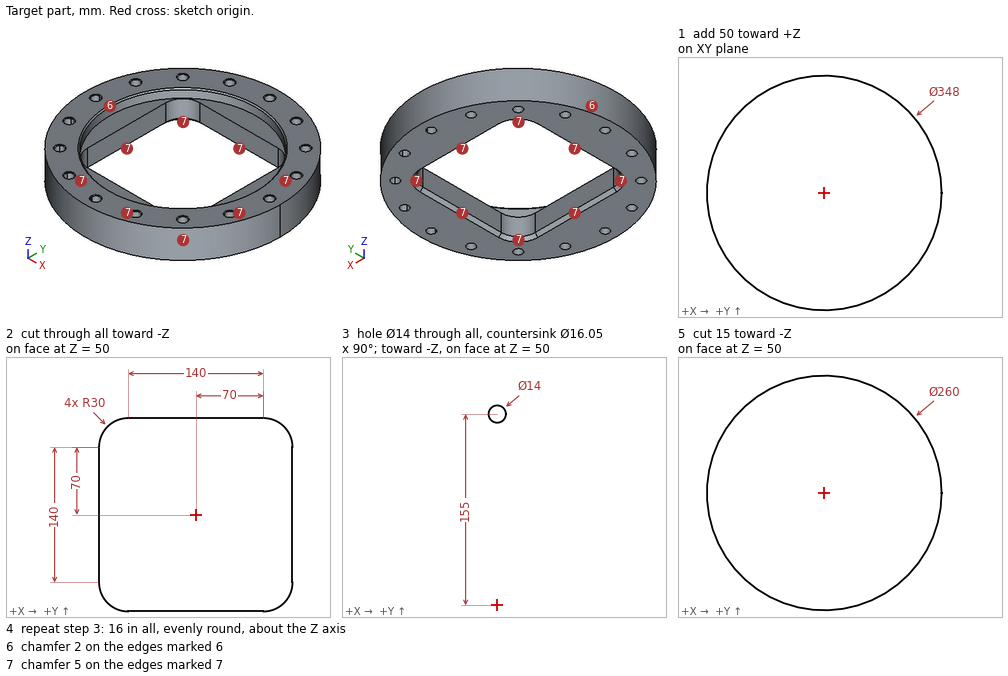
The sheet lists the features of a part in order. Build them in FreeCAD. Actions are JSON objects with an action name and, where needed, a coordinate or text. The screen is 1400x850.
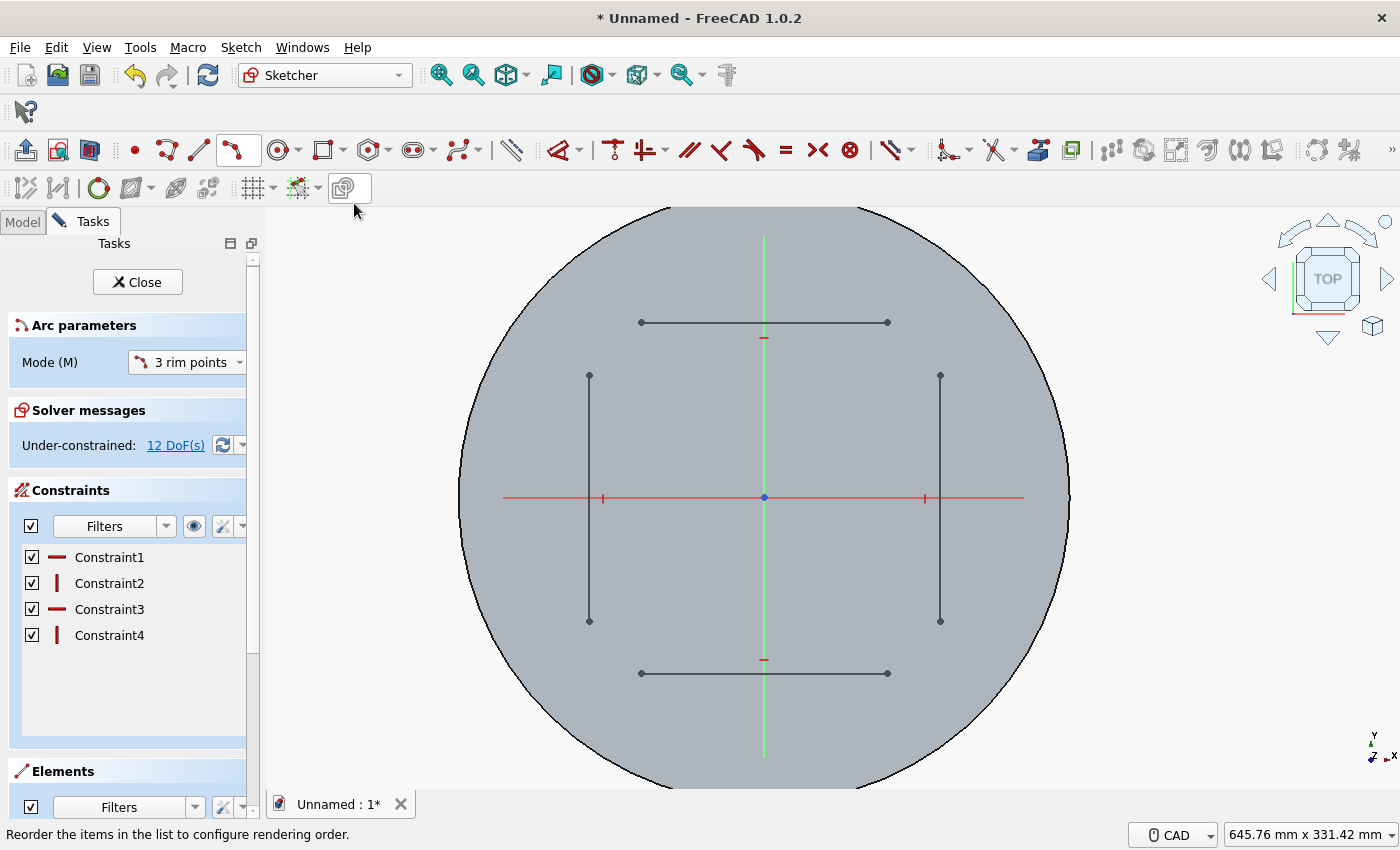
{"action": "left_click", "coordinate": [641, 323]}
{"action": "left_click", "coordinate": [589, 376]}
{"action": "left_click", "coordinate": [604, 338]}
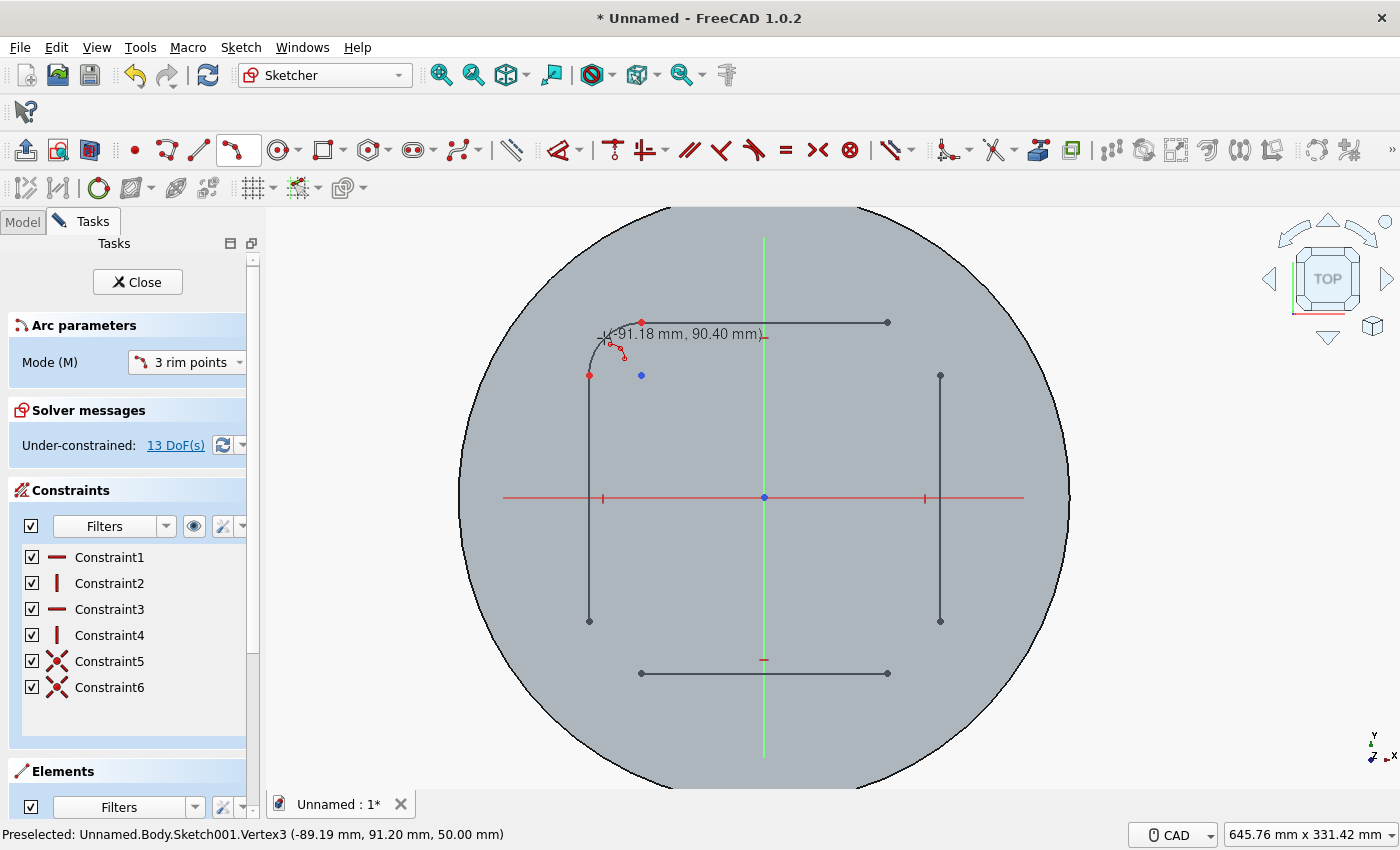
{"action": "left_click", "coordinate": [589, 622]}
{"action": "left_click", "coordinate": [641, 674]}
{"action": "left_click", "coordinate": [604, 658]}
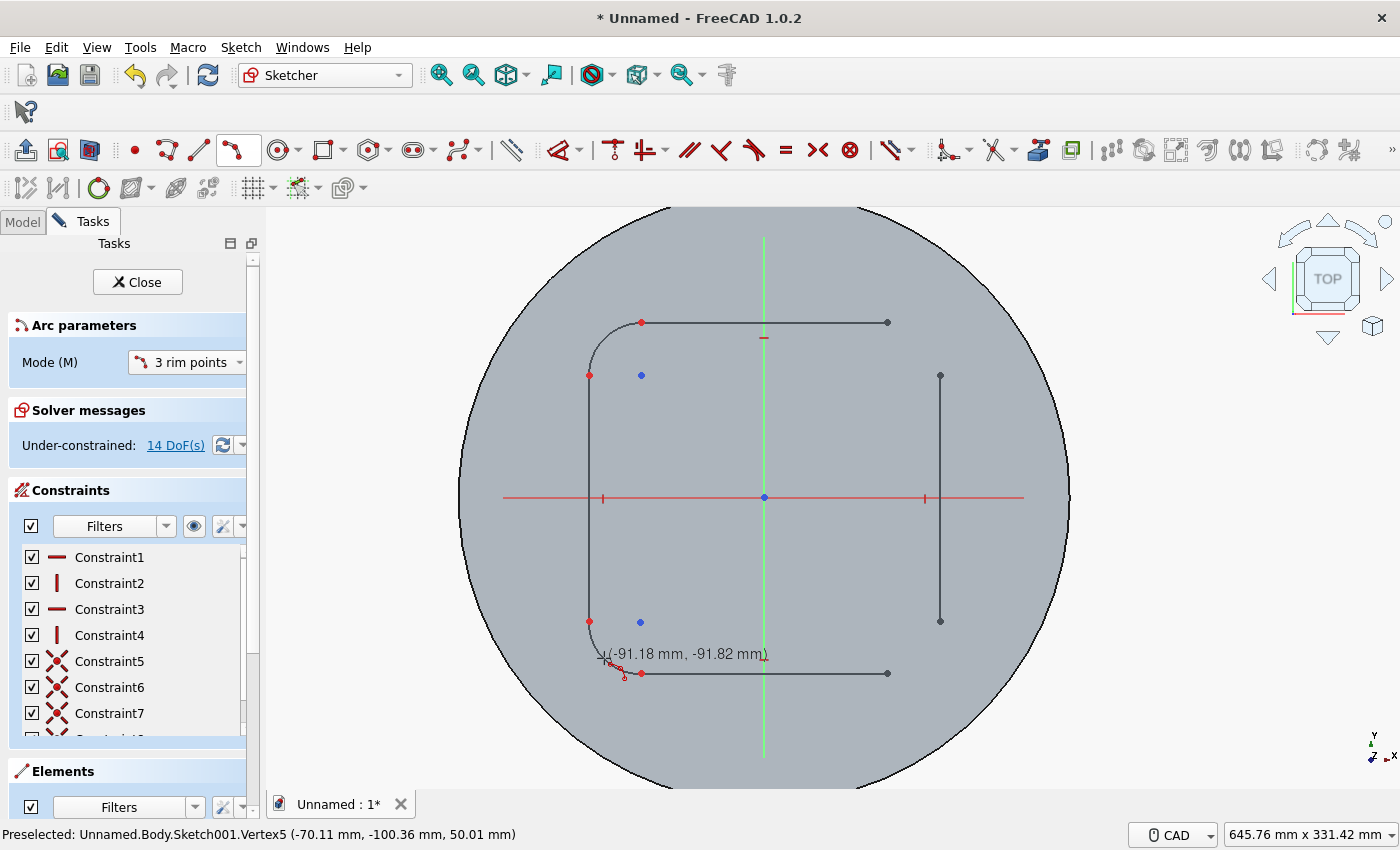
{"action": "left_click", "coordinate": [887, 674]}
{"action": "left_click", "coordinate": [940, 622]}
{"action": "left_click", "coordinate": [924, 658]}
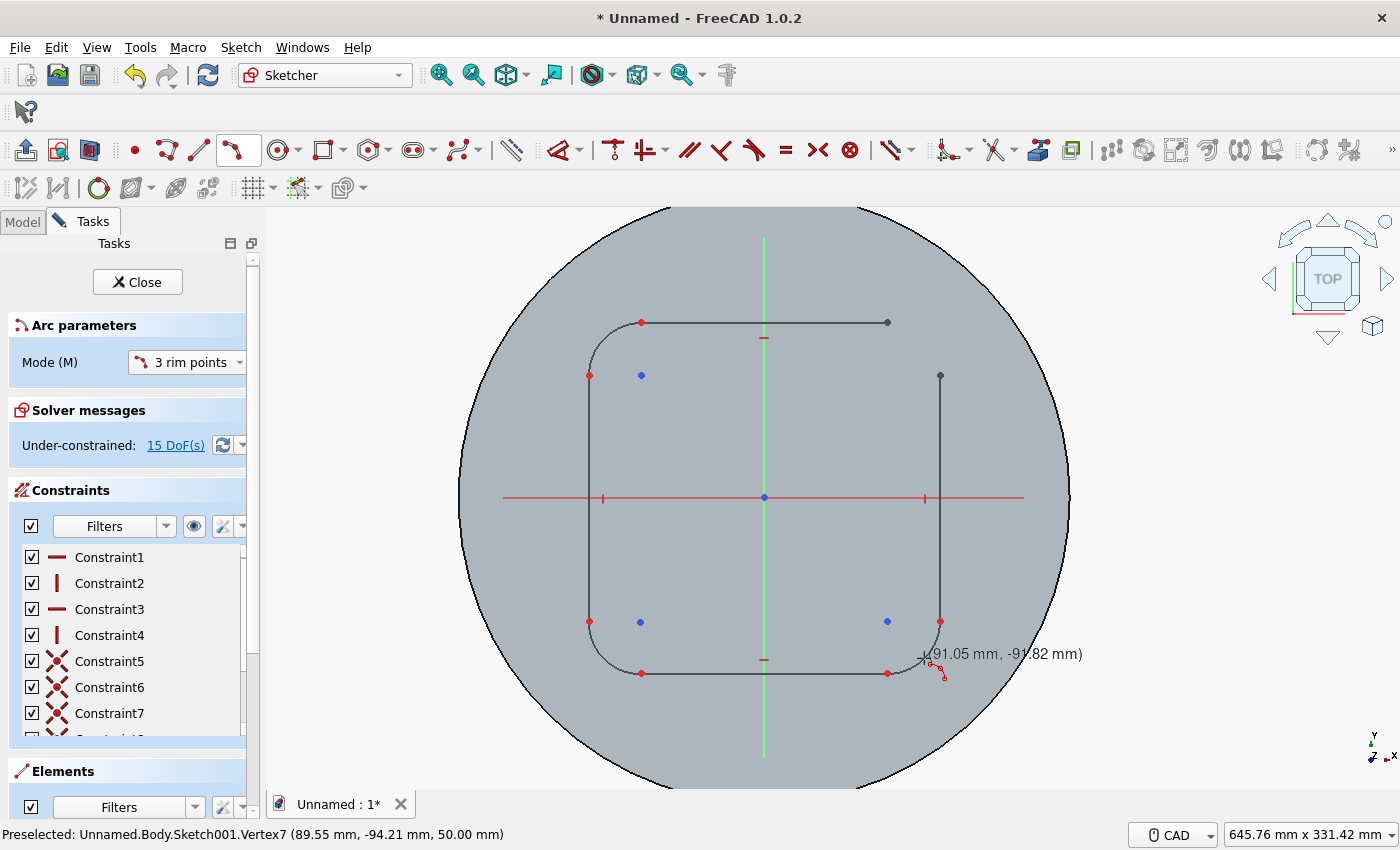
{"action": "left_click", "coordinate": [940, 376]}
{"action": "left_click", "coordinate": [887, 323]}
{"action": "left_click", "coordinate": [924, 338]}
{"action": "key", "text": "Escape"}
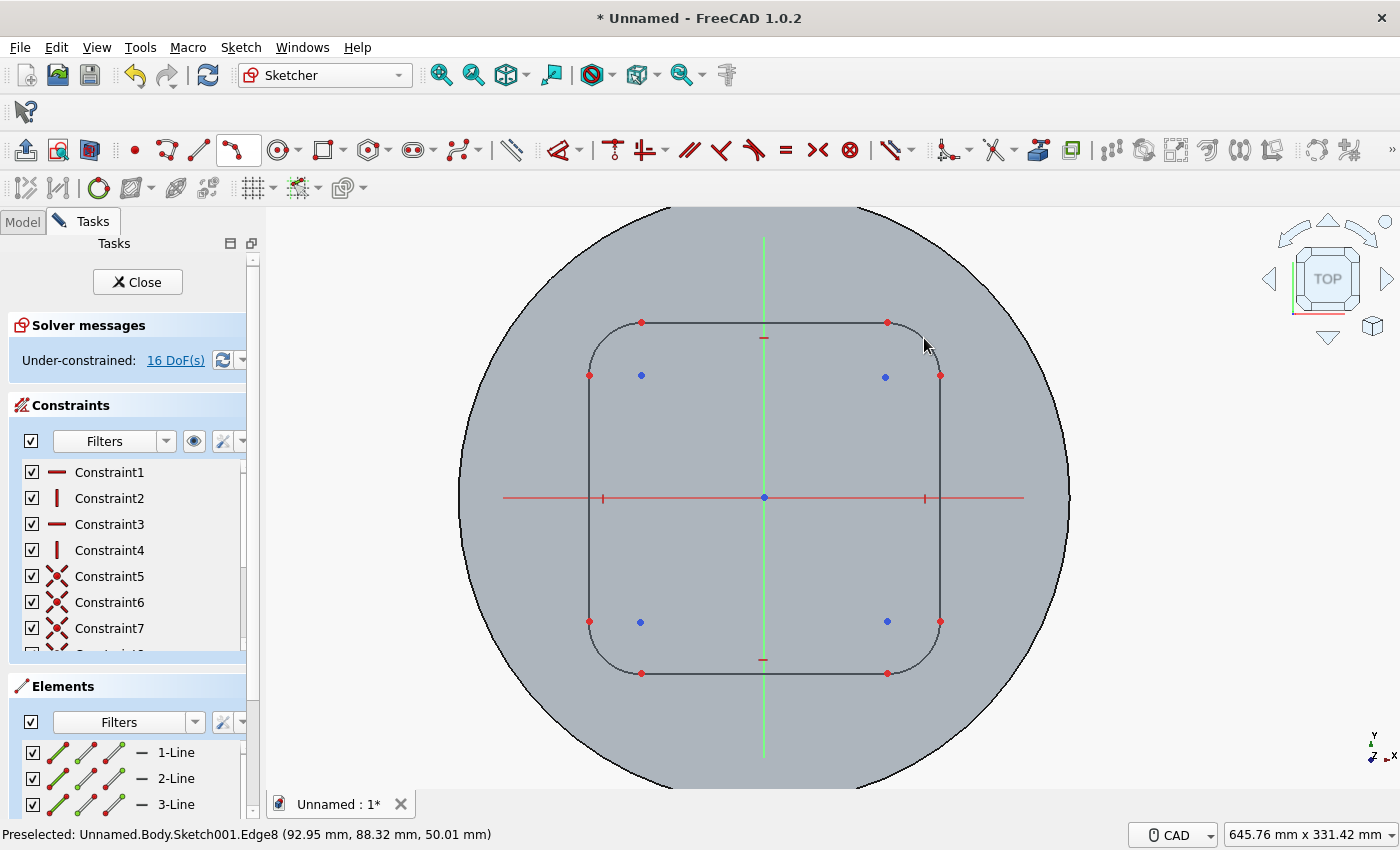
{"action": "left_click", "coordinate": [813, 323]}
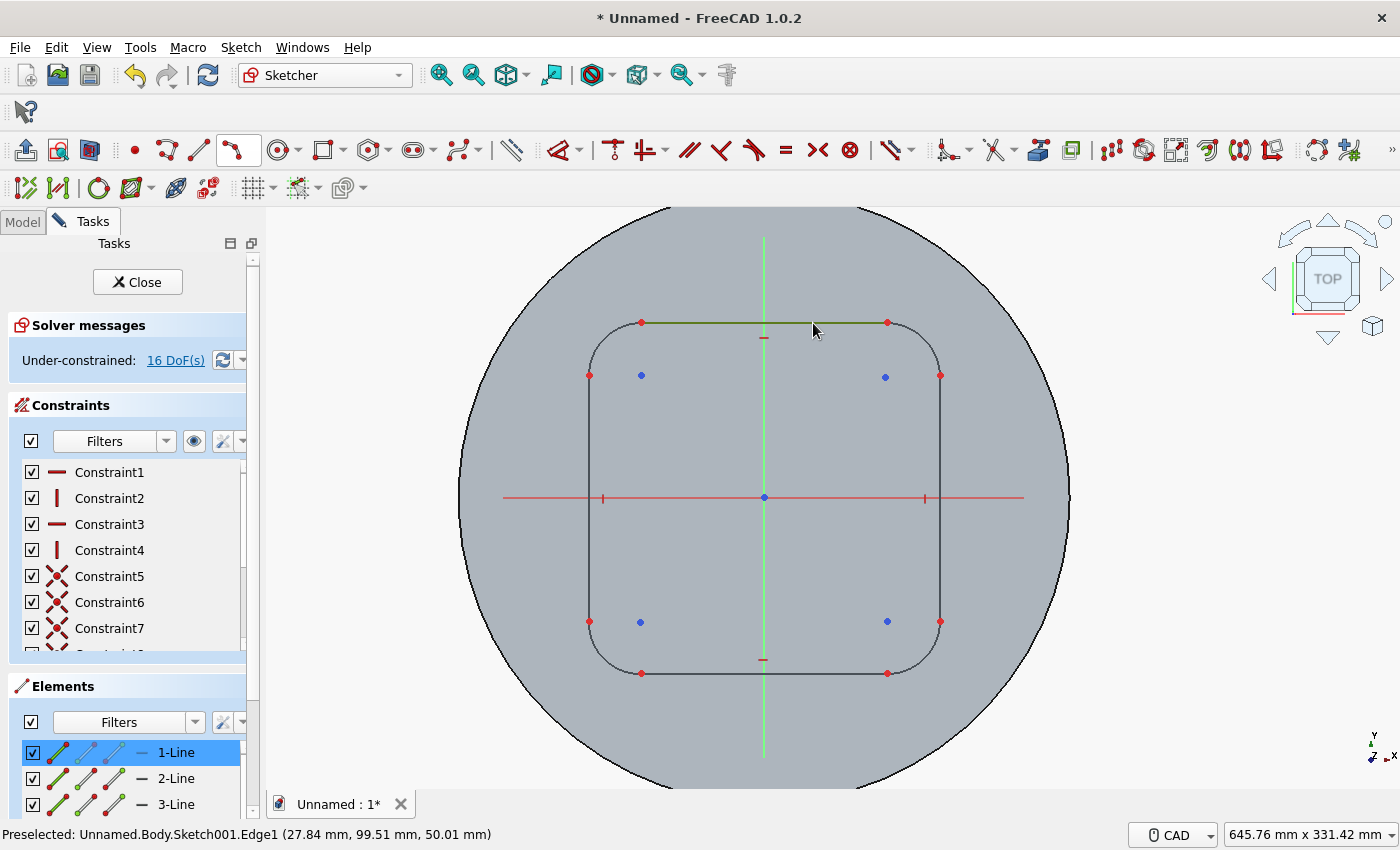
{"action": "left_click", "coordinate": [617, 329]}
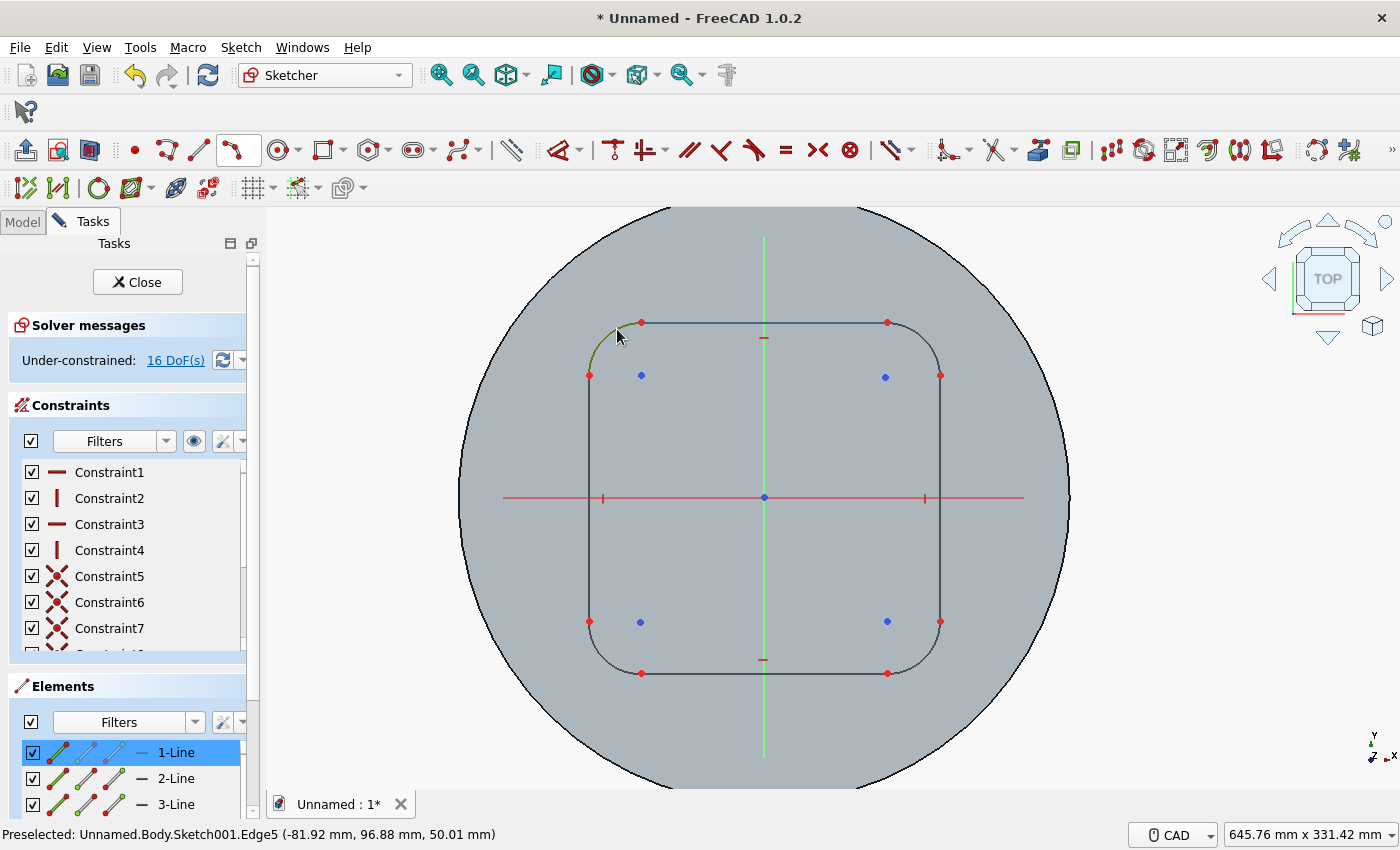
{"action": "left_click", "coordinate": [754, 150]}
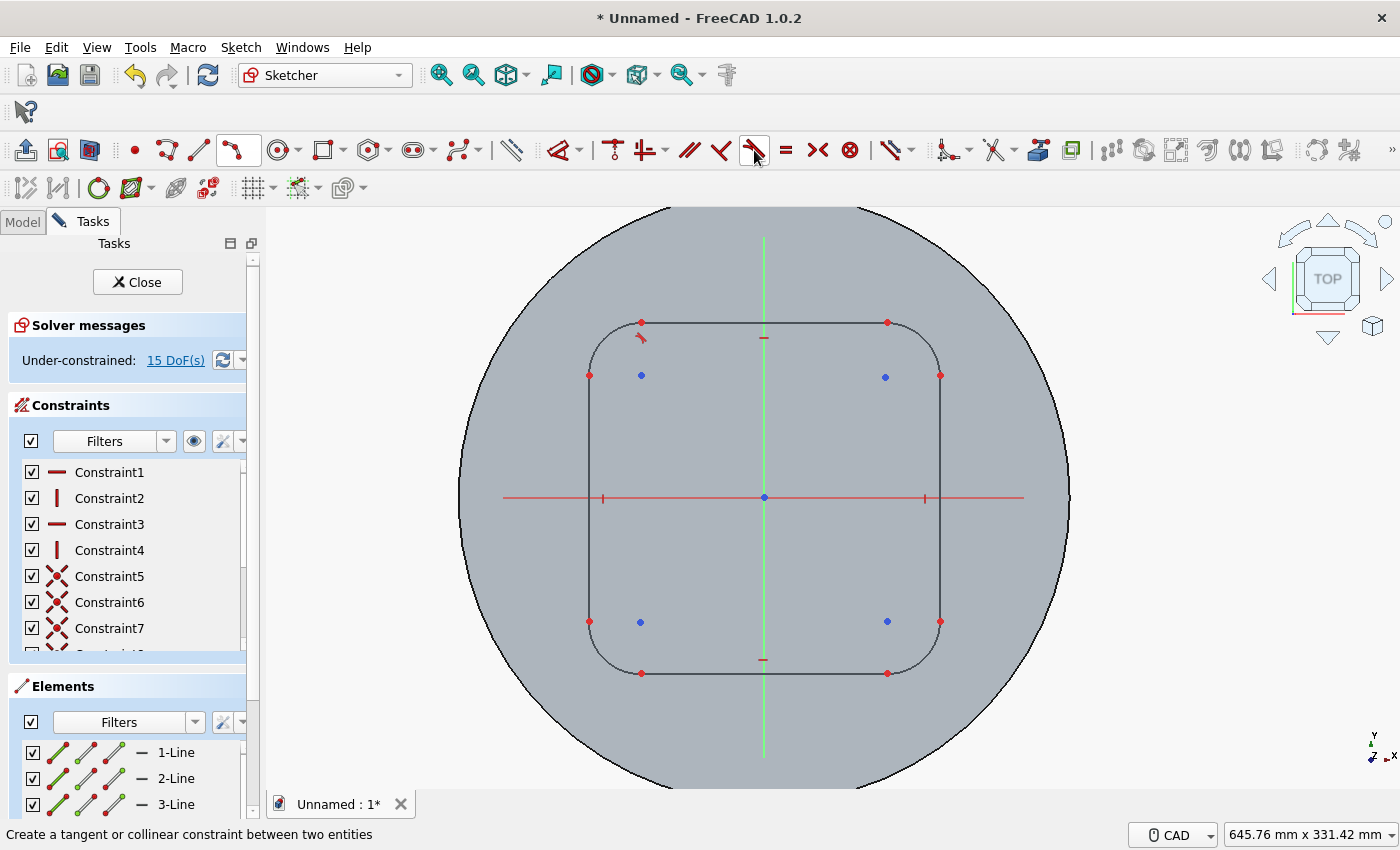
{"action": "left_click", "coordinate": [813, 323]}